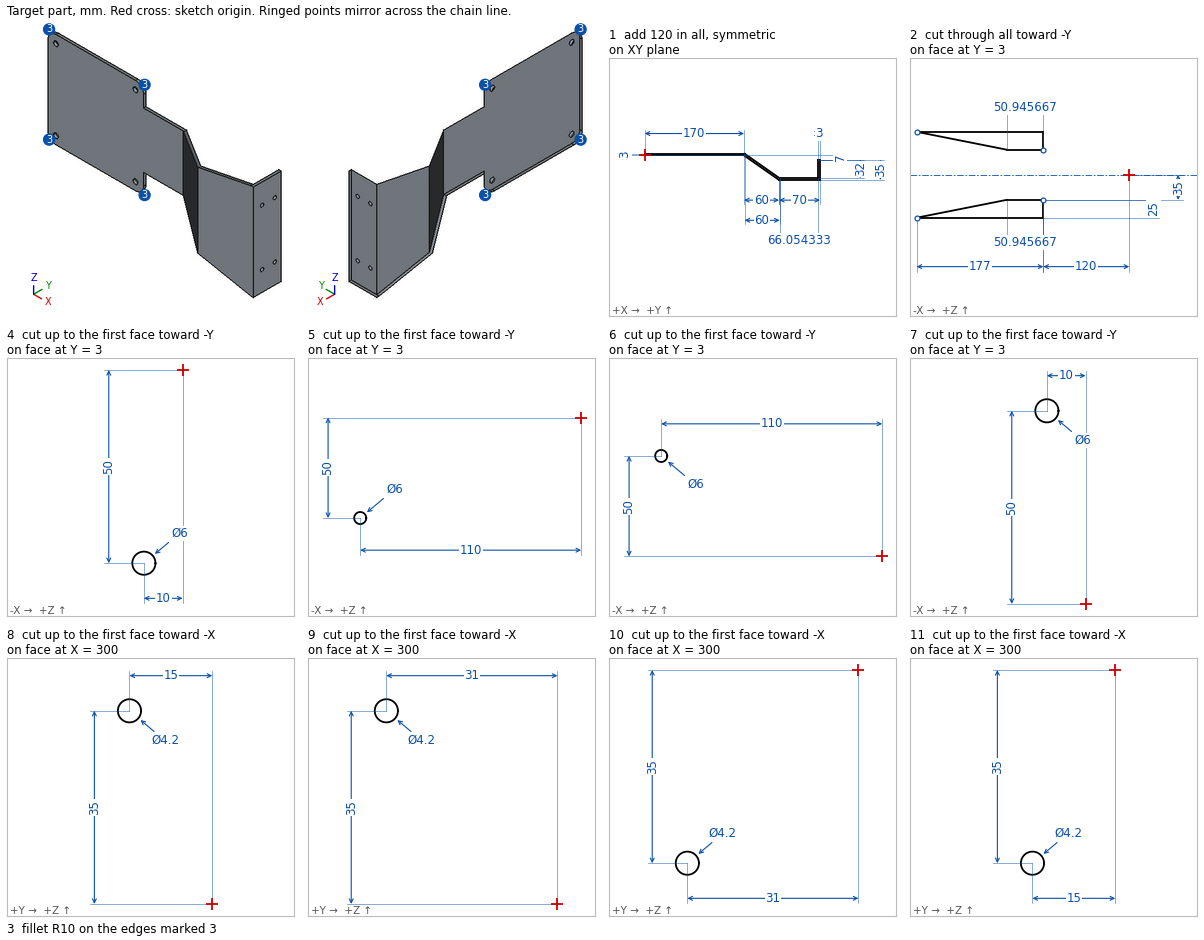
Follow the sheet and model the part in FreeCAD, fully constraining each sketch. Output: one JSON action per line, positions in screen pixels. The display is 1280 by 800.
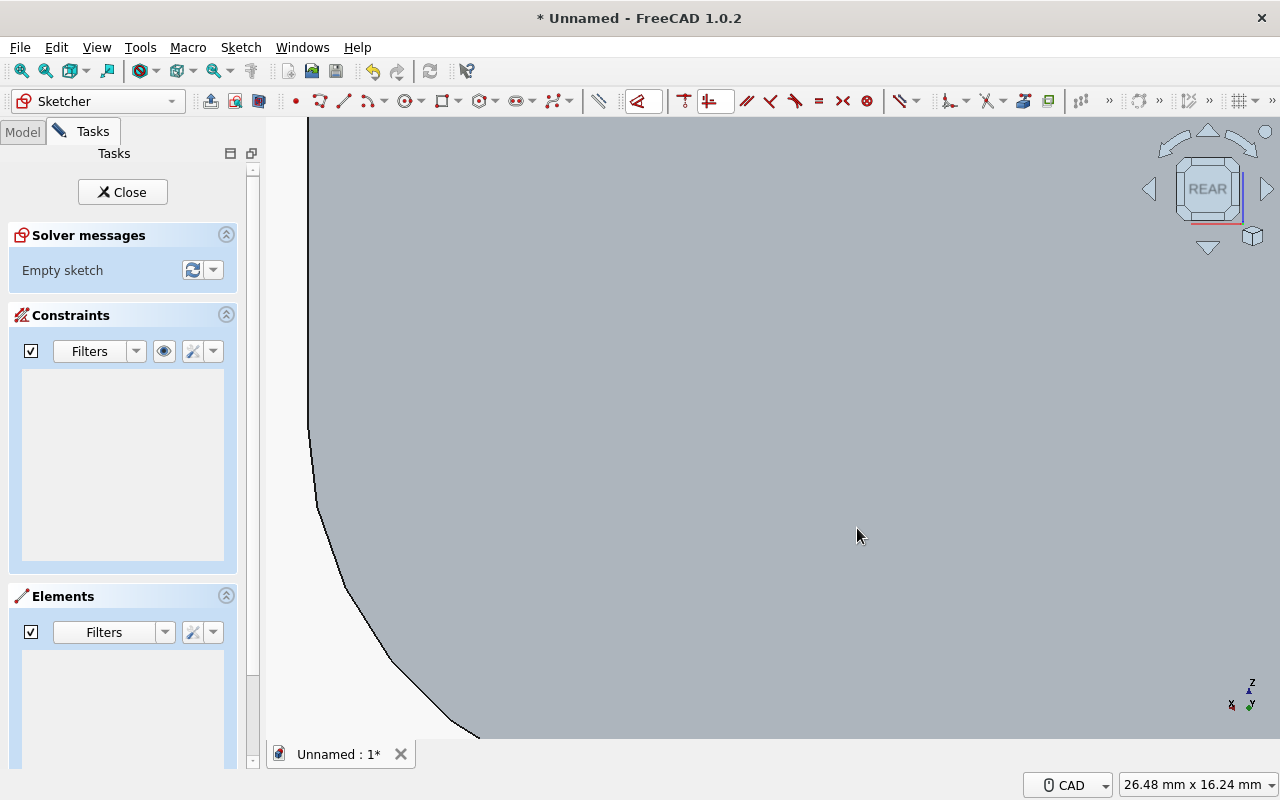
{"action": "scroll", "coordinate": [674, 414], "scroll_direction": "up", "scroll_amount": 3}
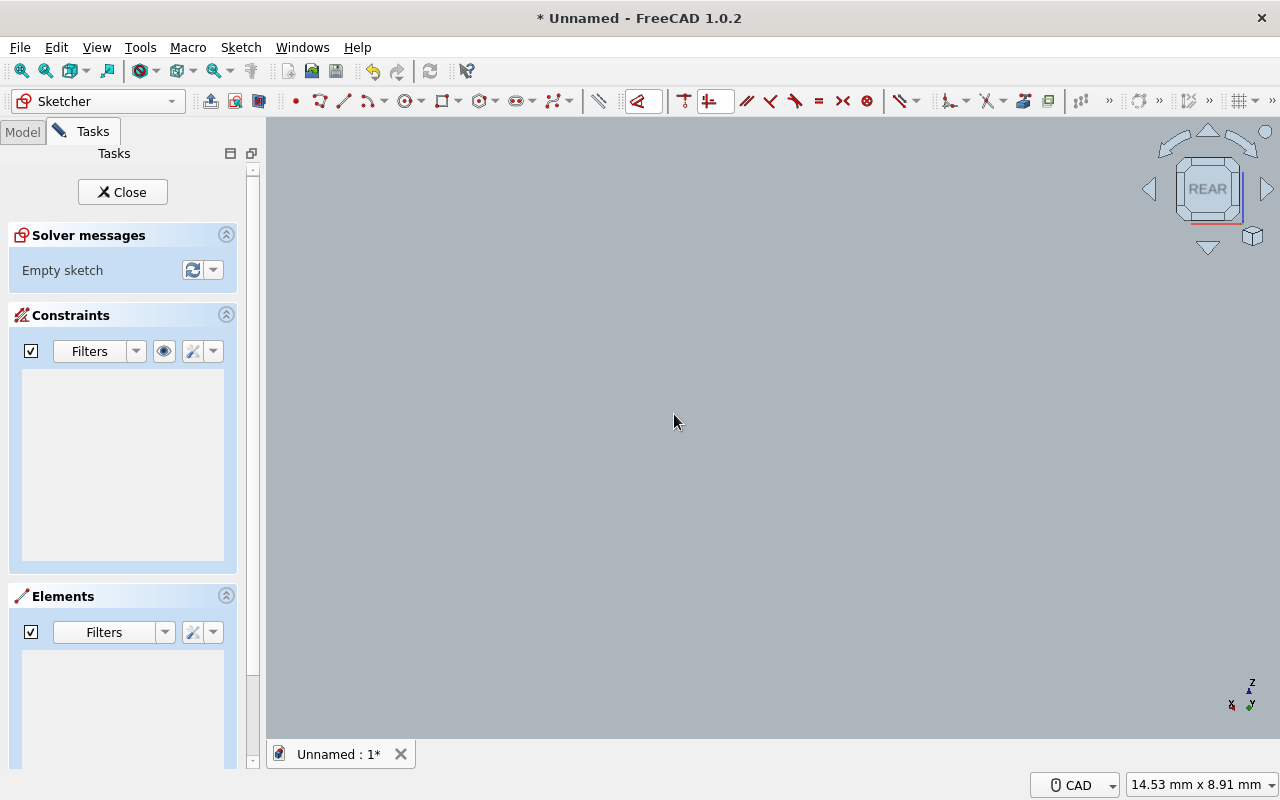
{"action": "left_click", "coordinate": [406, 102]}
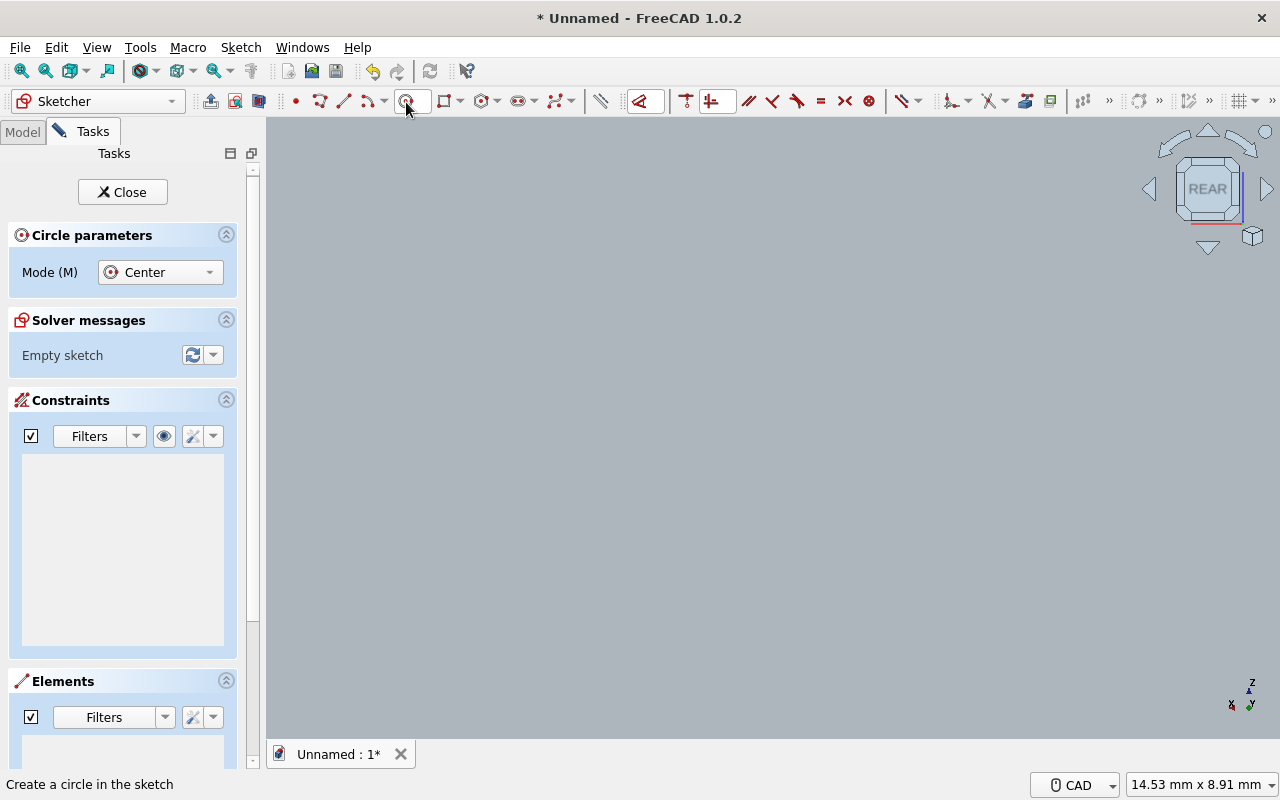
{"action": "left_click", "coordinate": [704, 427]}
{"action": "left_click", "coordinate": [852, 279]}
{"action": "key", "text": "Escape"}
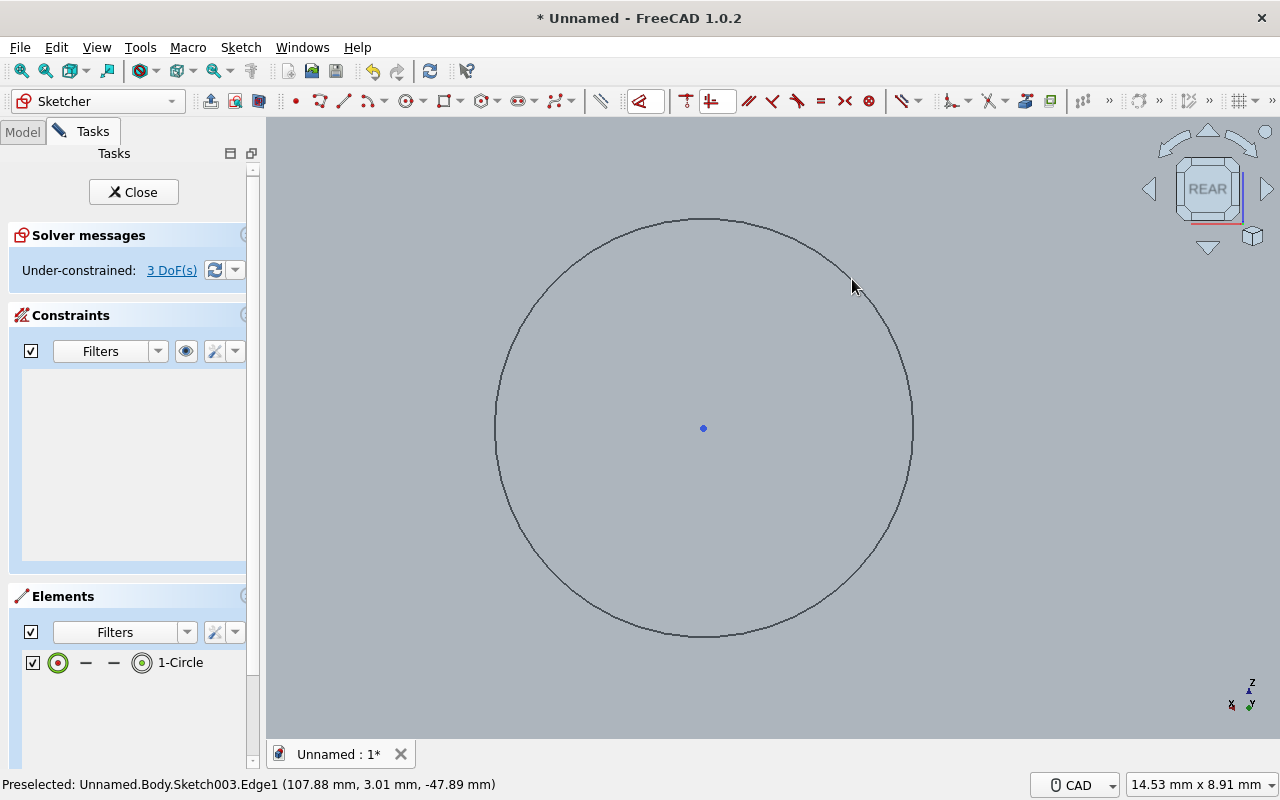
{"action": "left_click", "coordinate": [852, 280]}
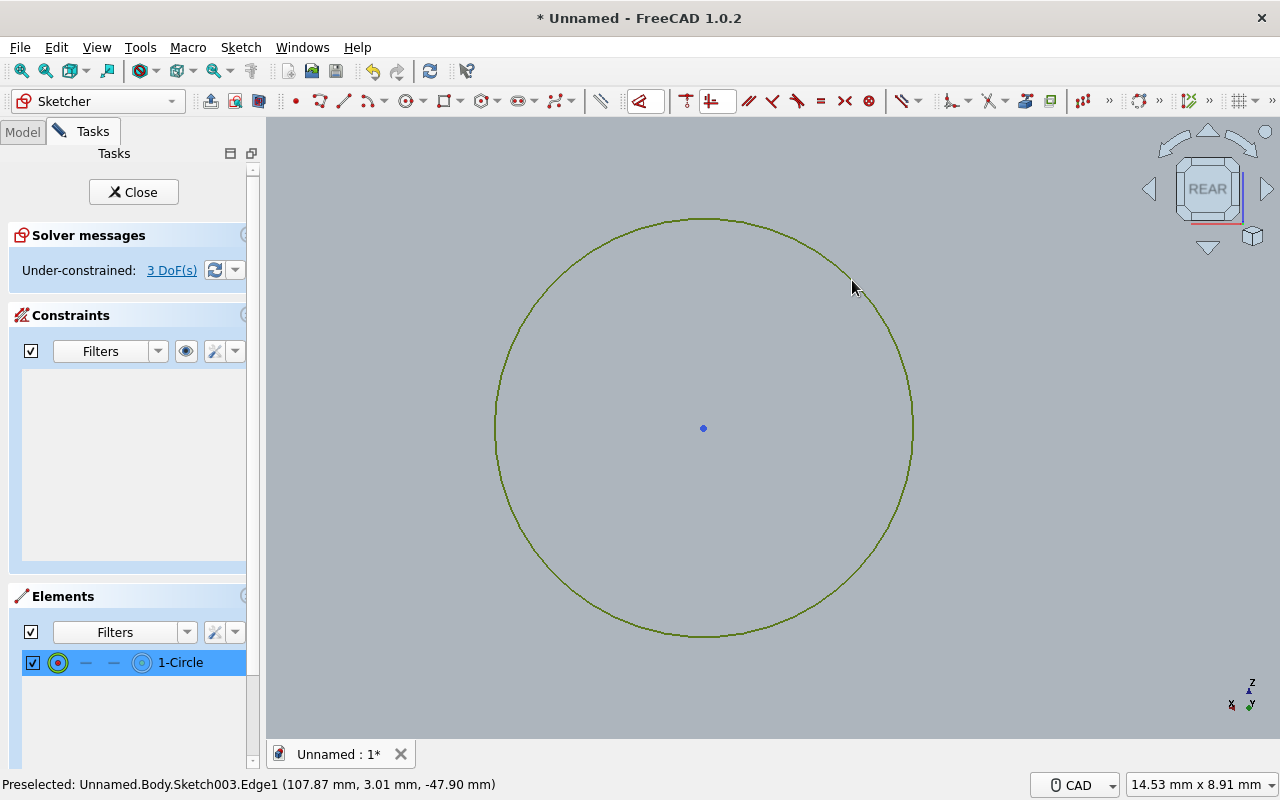
{"action": "left_click", "coordinate": [658, 102]}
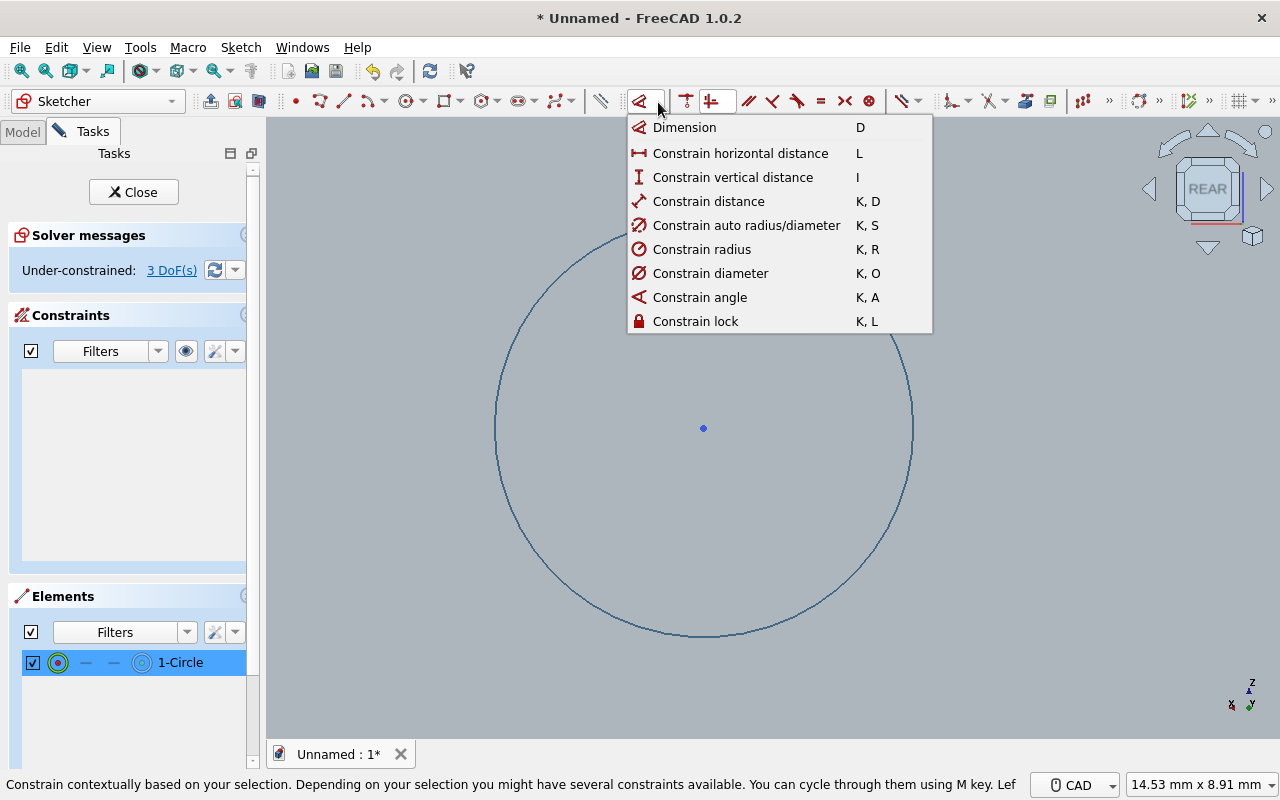
{"action": "left_click", "coordinate": [780, 273]}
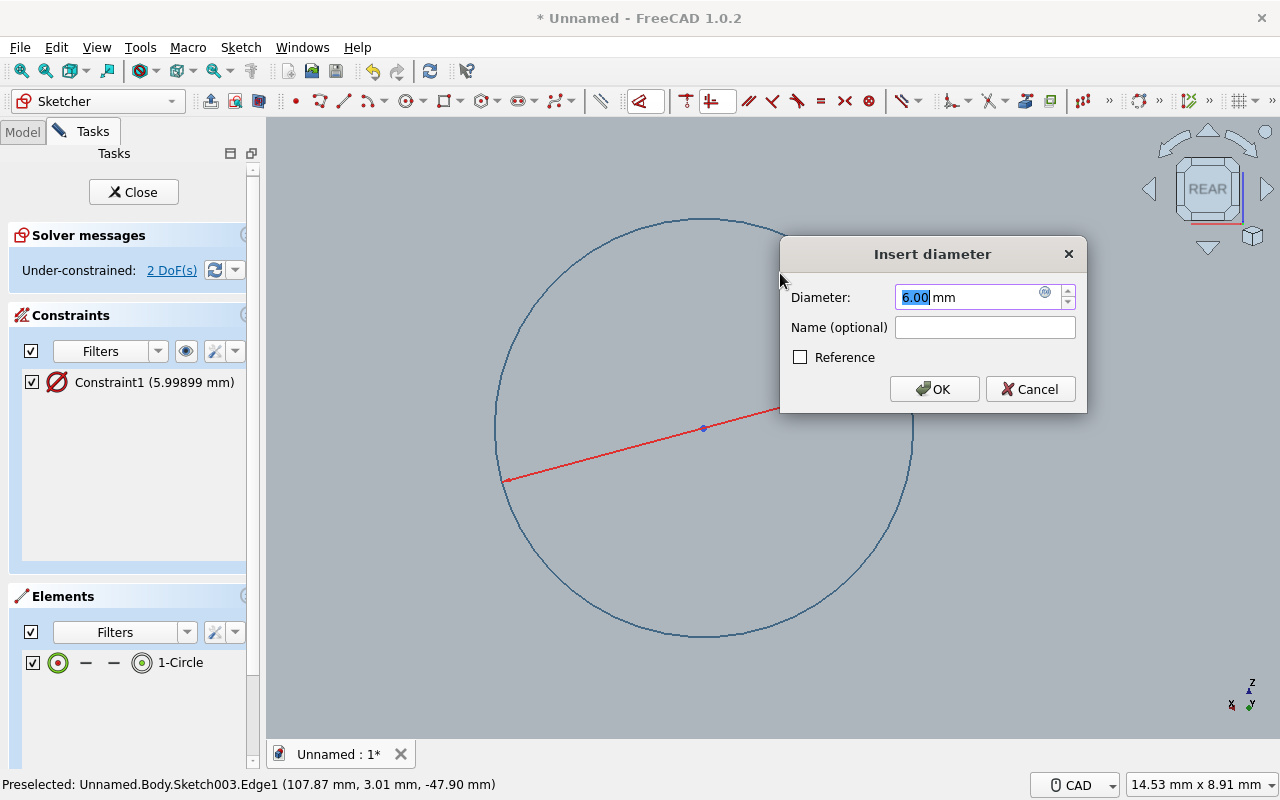
{"action": "type", "text": "6"}
{"action": "key", "text": "Return"}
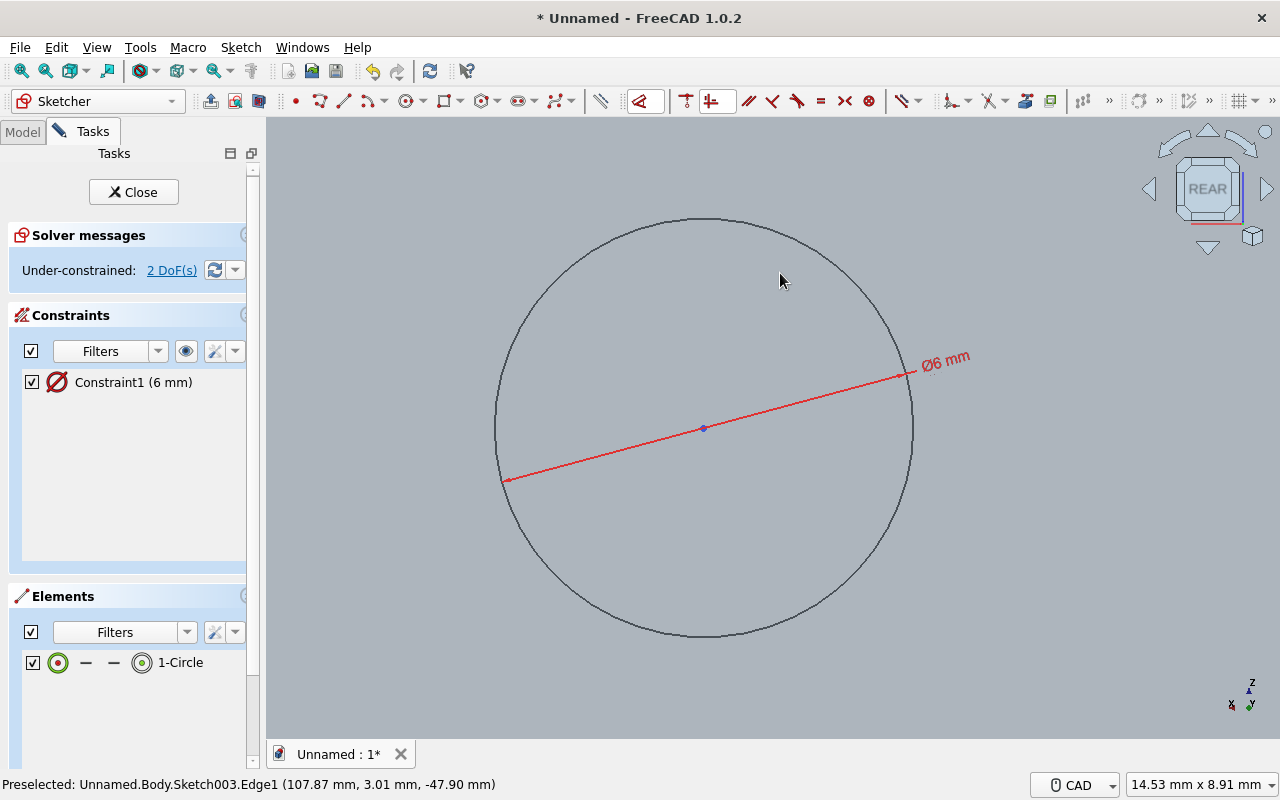
{"action": "left_click", "coordinate": [704, 428]}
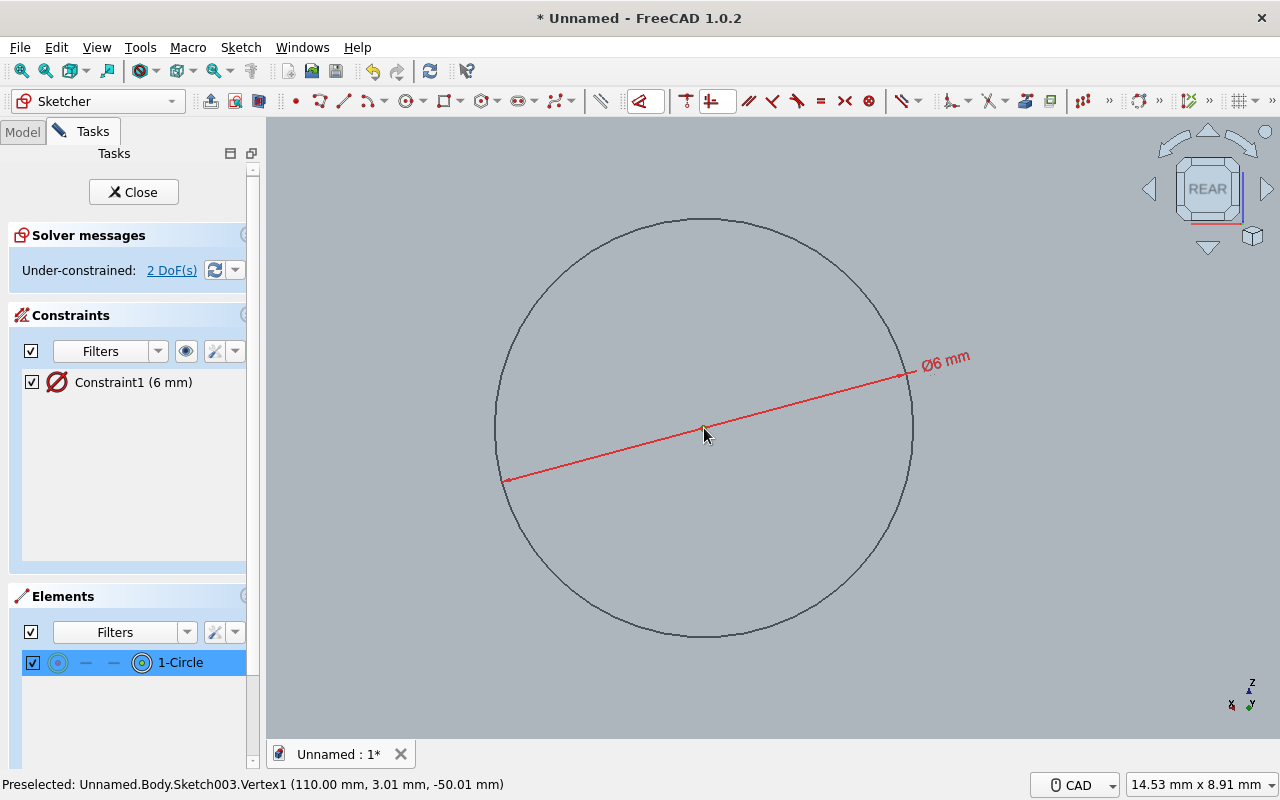
{"action": "left_click", "coordinate": [658, 102]}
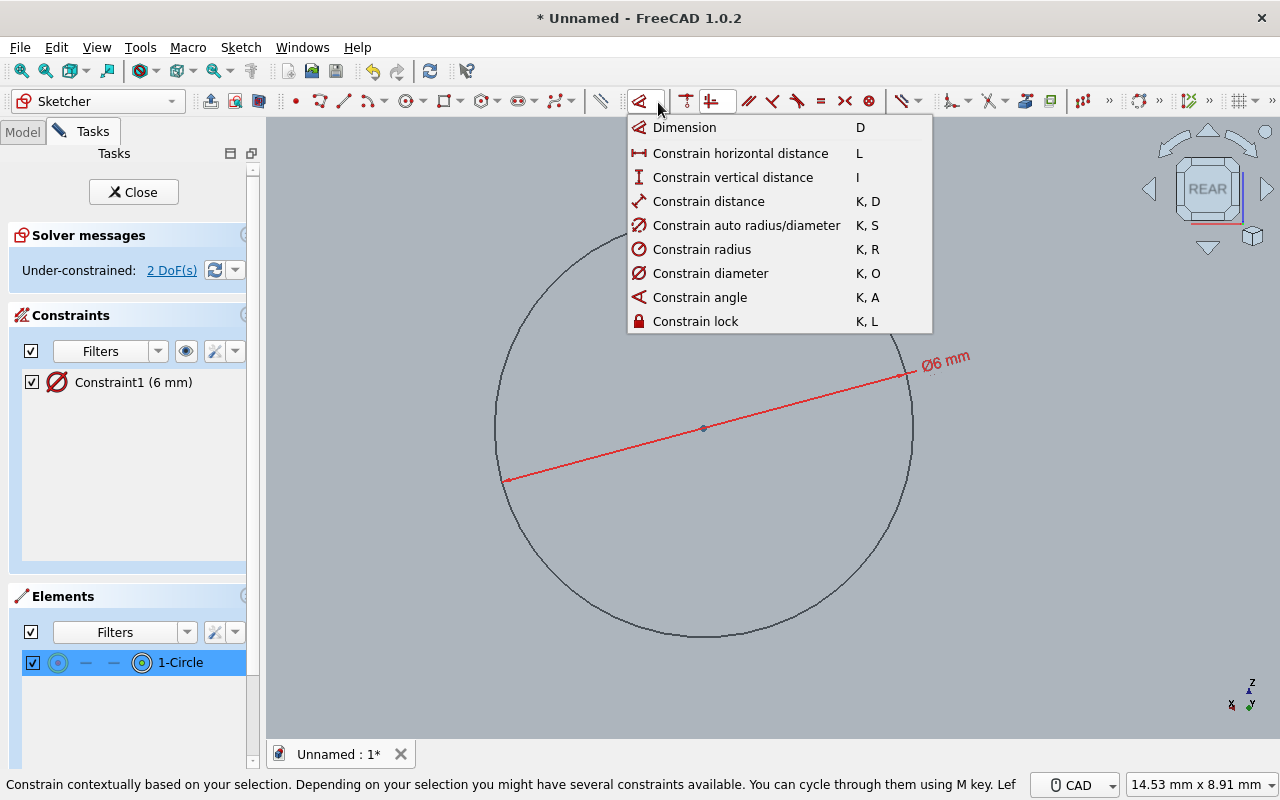
{"action": "left_click", "coordinate": [780, 177]}